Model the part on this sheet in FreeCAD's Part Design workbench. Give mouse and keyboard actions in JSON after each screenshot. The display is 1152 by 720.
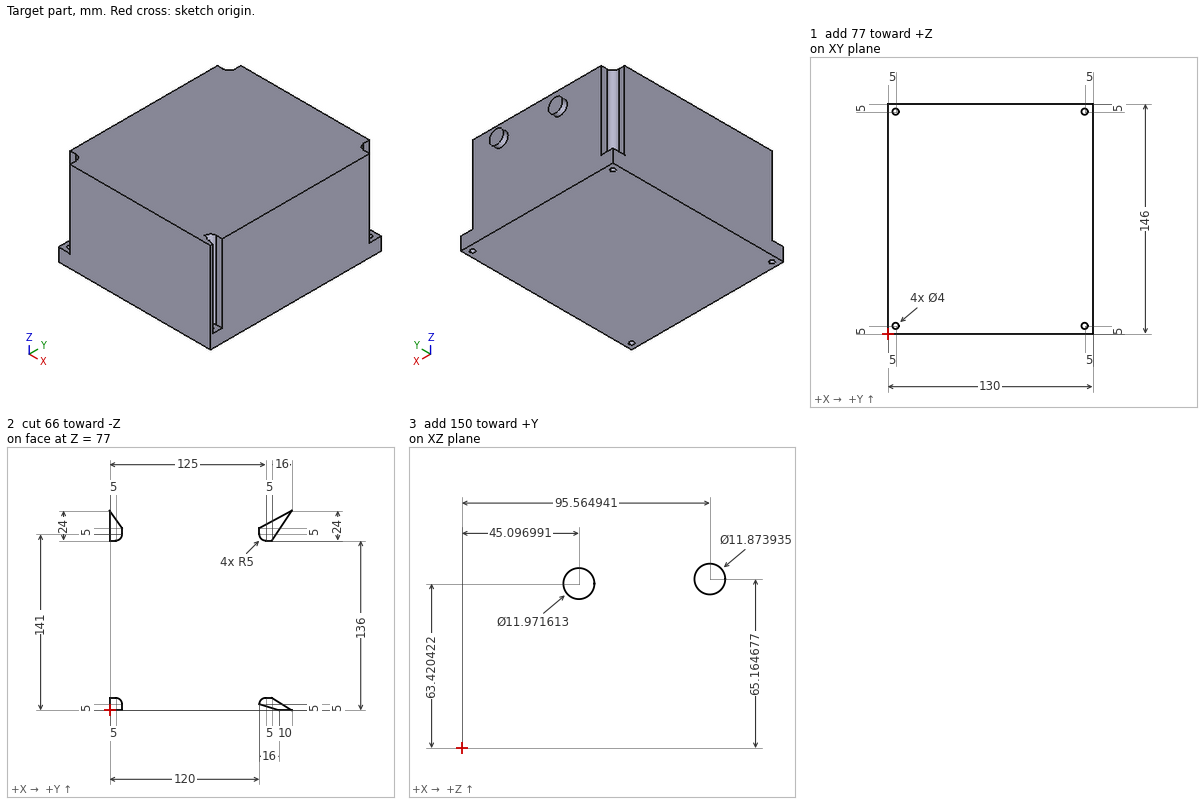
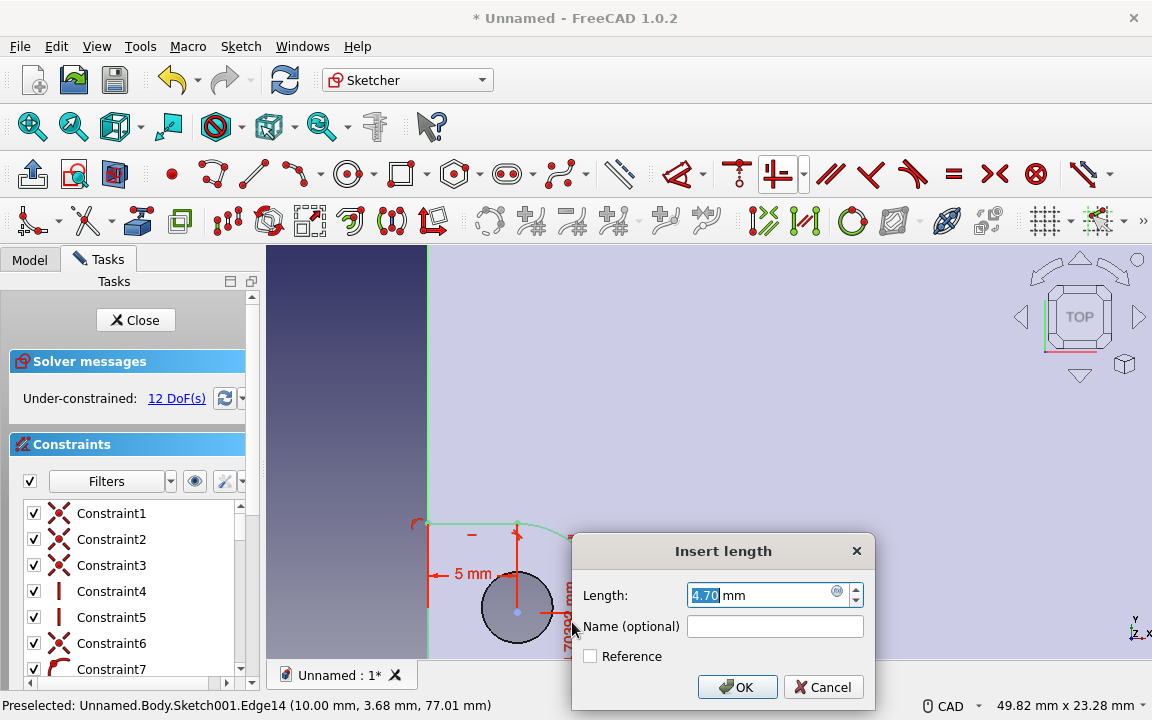
{"action": "type", "text": "5"}
{"action": "key", "text": "Return"}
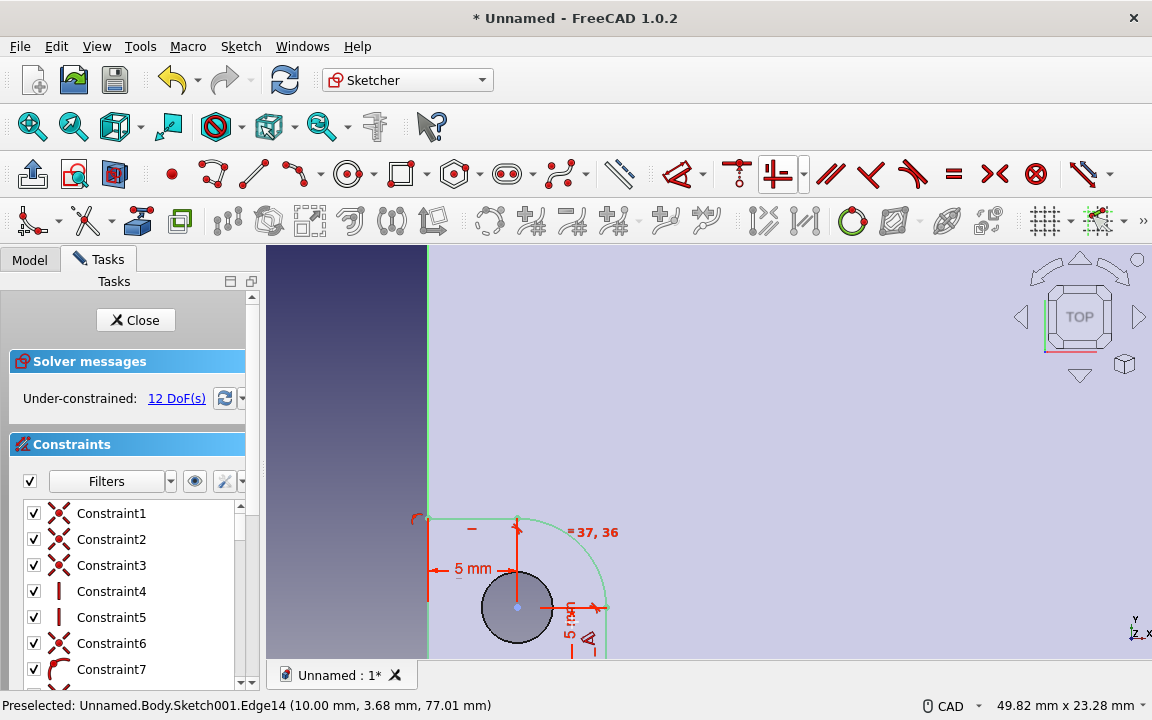
{"action": "scroll", "coordinate": [532, 570], "scroll_direction": "down", "scroll_amount": 12}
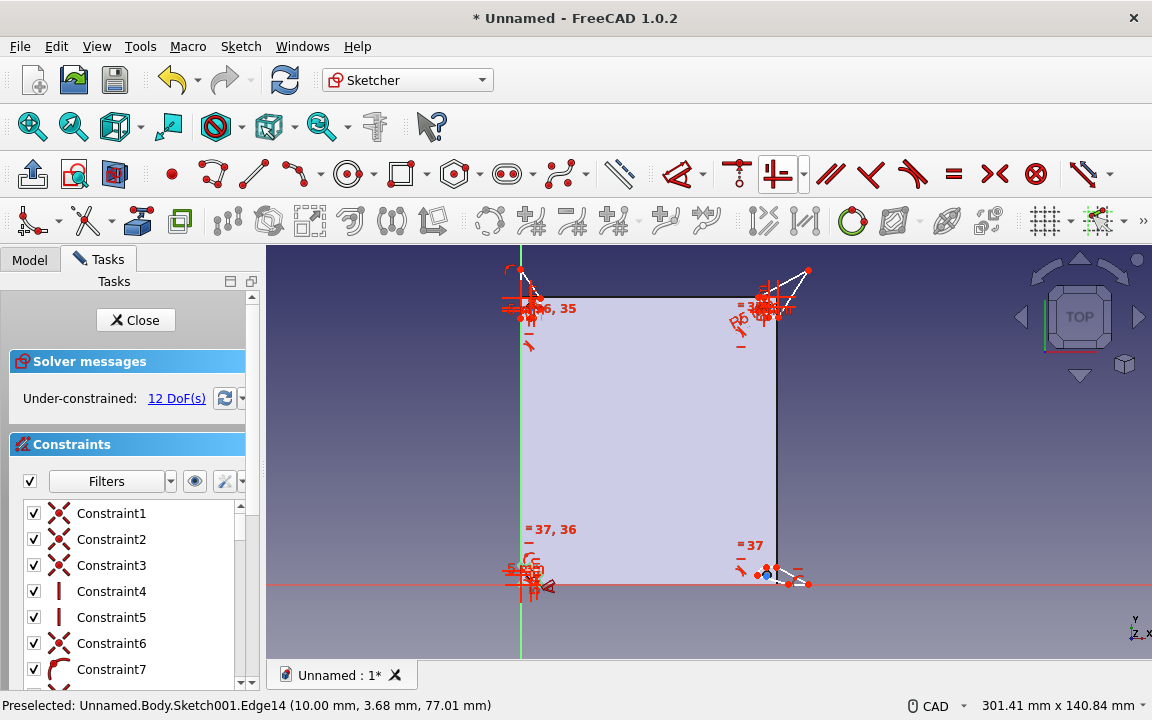
{"action": "scroll", "coordinate": [730, 568], "scroll_direction": "up", "scroll_amount": 9}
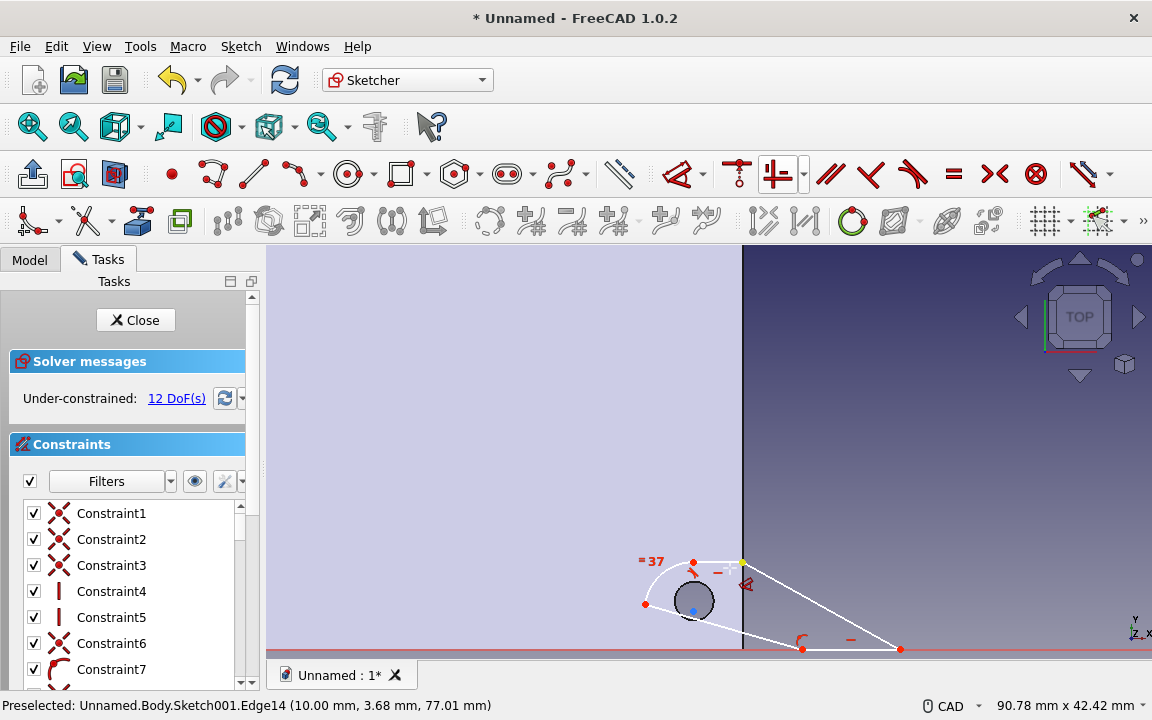
{"action": "left_click", "coordinate": [728, 562]}
{"action": "left_click", "coordinate": [718, 596]}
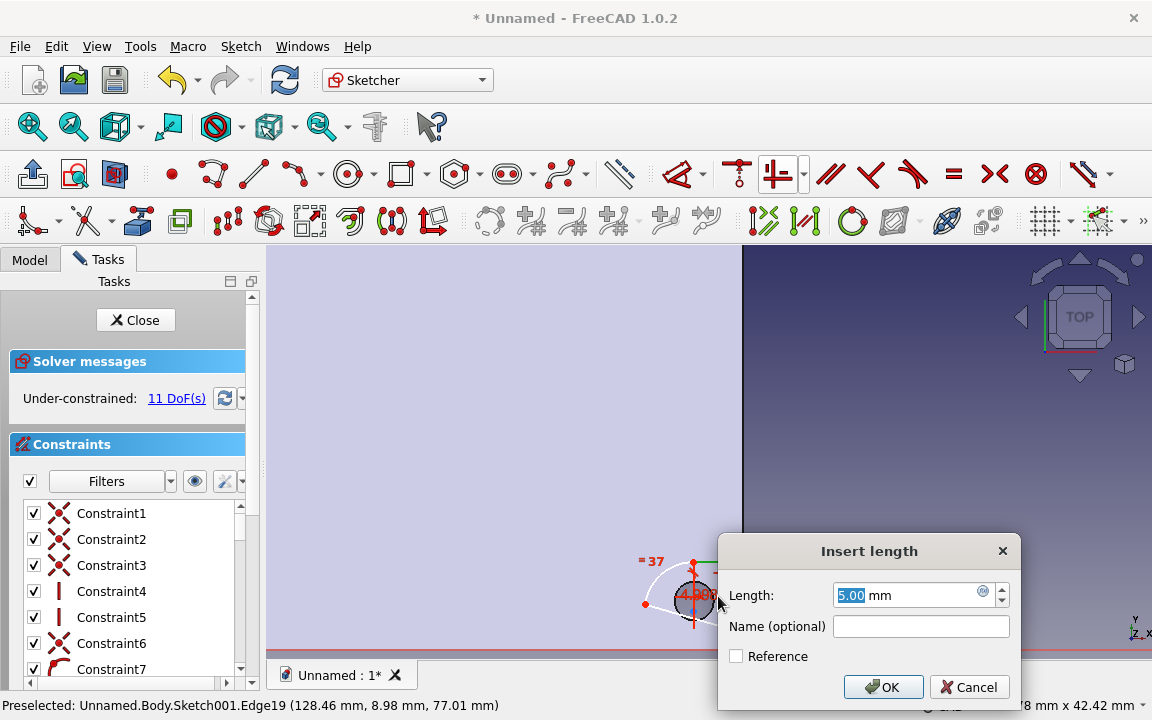
{"action": "type", "text": "5"}
{"action": "key", "text": "Return"}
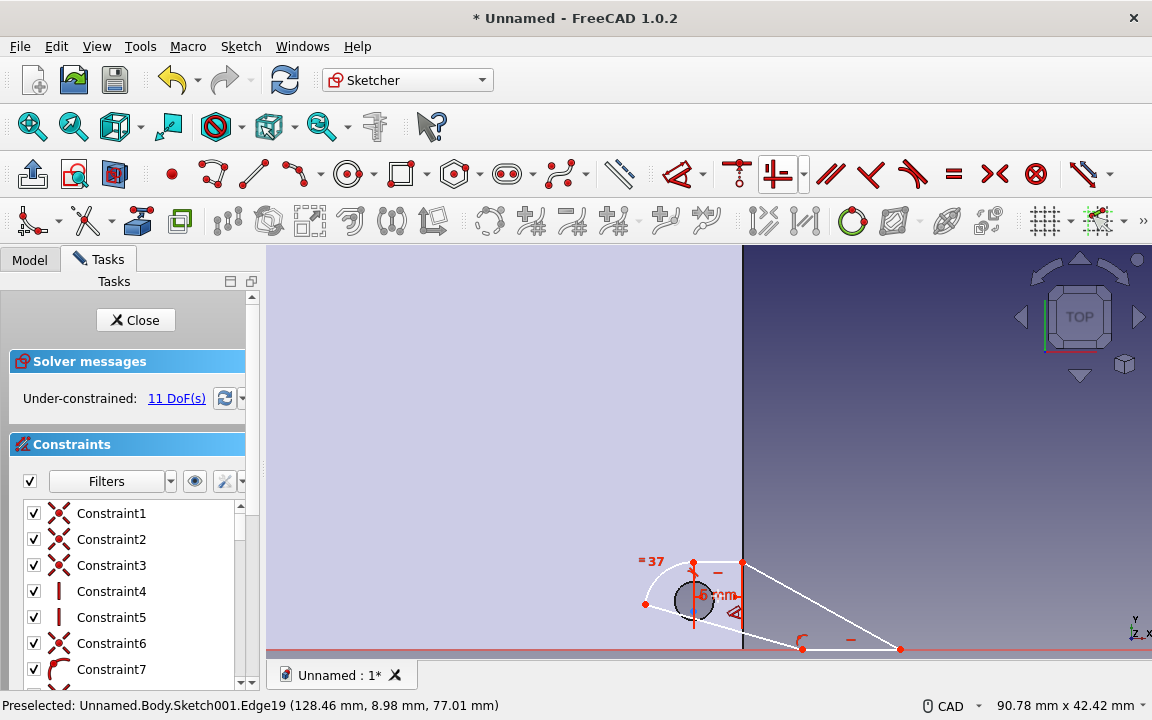
{"action": "scroll", "coordinate": [730, 567], "scroll_direction": "down", "scroll_amount": 9}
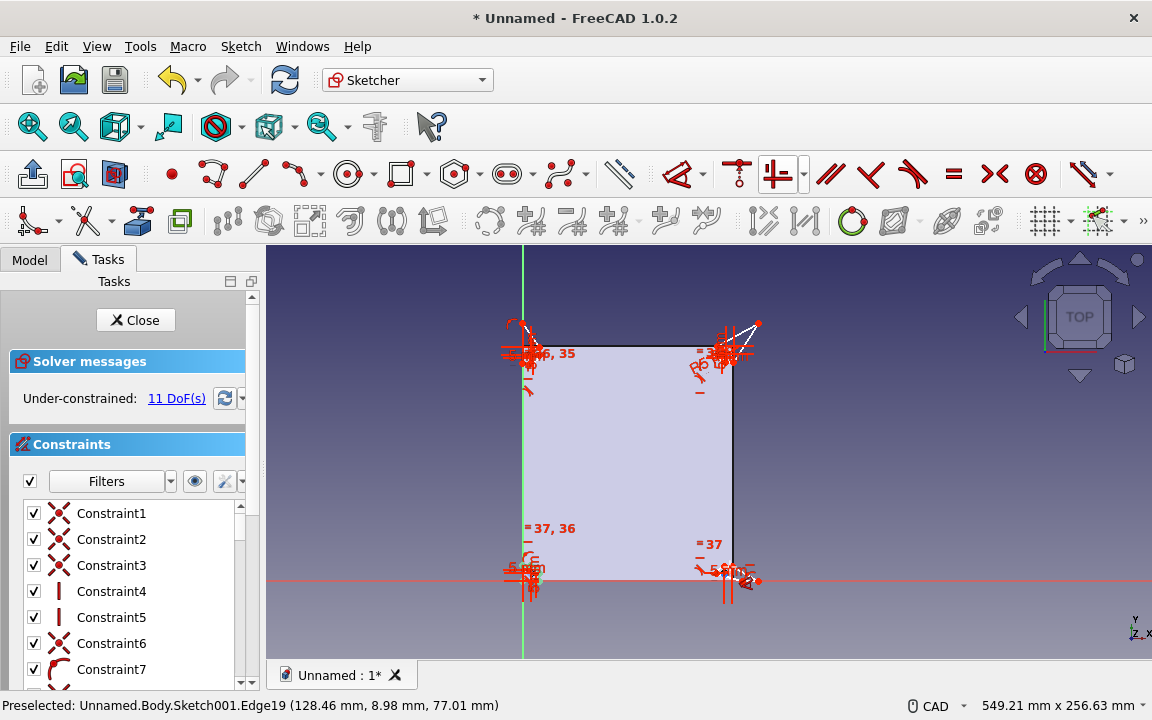
{"action": "scroll", "coordinate": [523, 335], "scroll_direction": "up", "scroll_amount": 4}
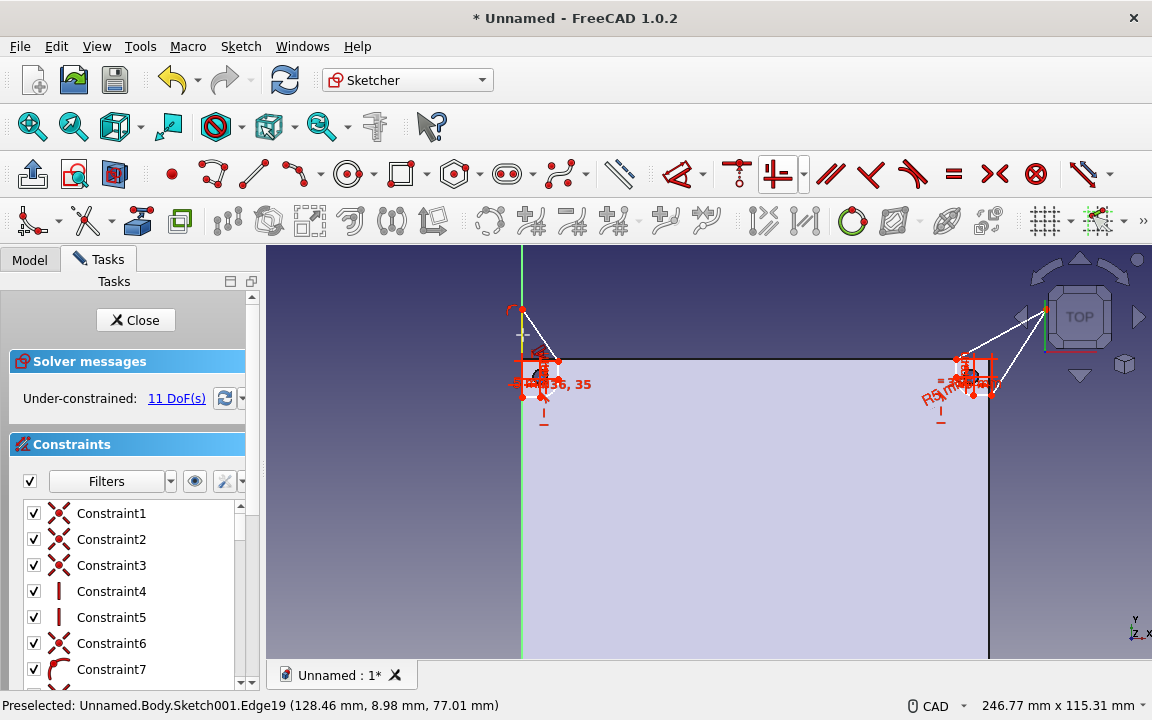
{"action": "left_click", "coordinate": [522, 336]}
{"action": "left_click", "coordinate": [488, 333]}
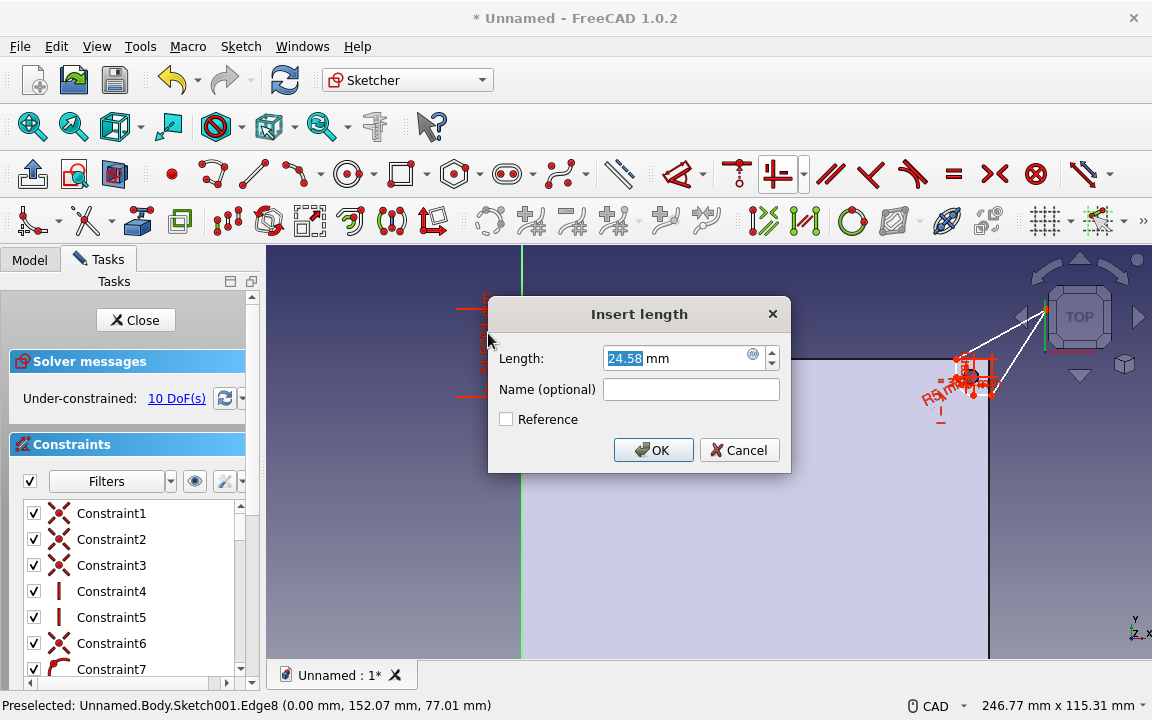
{"action": "type", "text": "24"}
{"action": "key", "text": "Return"}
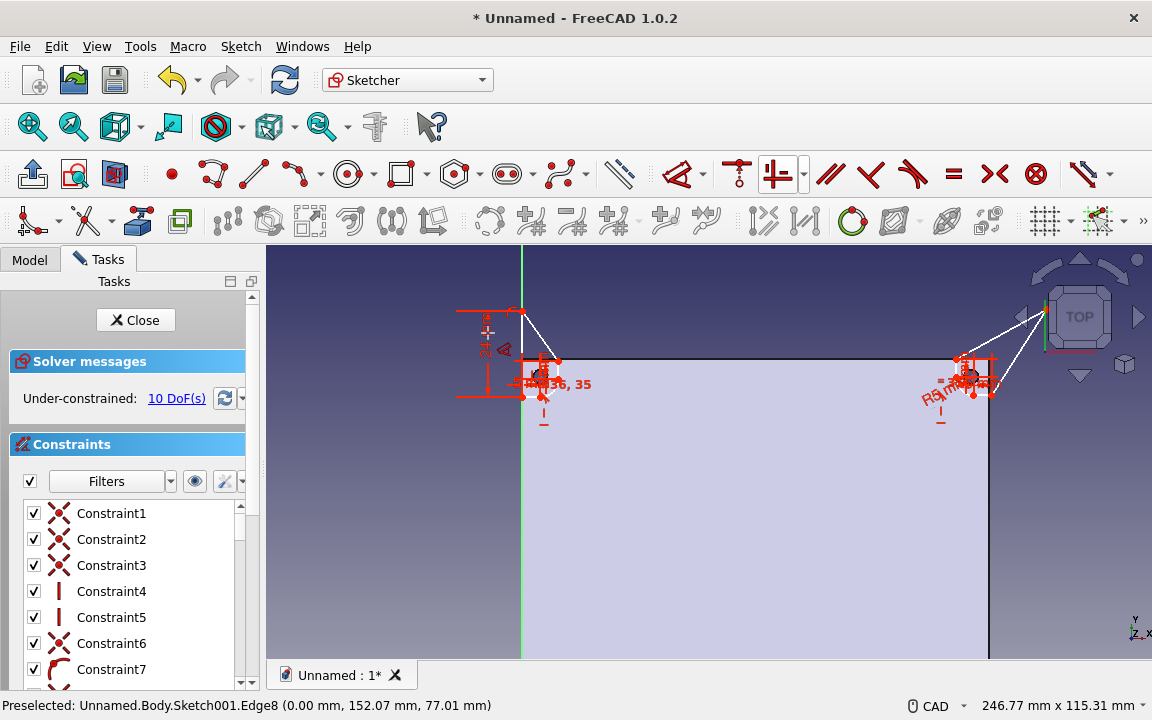
{"action": "scroll", "coordinate": [523, 335], "scroll_direction": "down", "scroll_amount": 4}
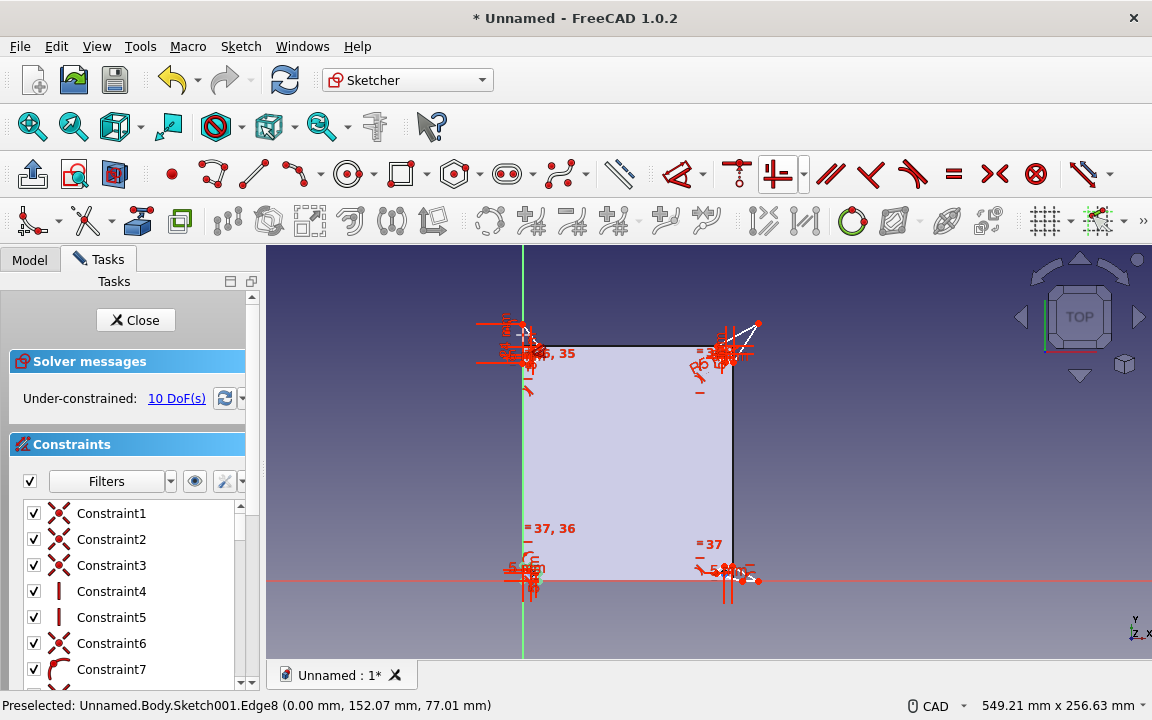
{"action": "scroll", "coordinate": [747, 581], "scroll_direction": "up", "scroll_amount": 6}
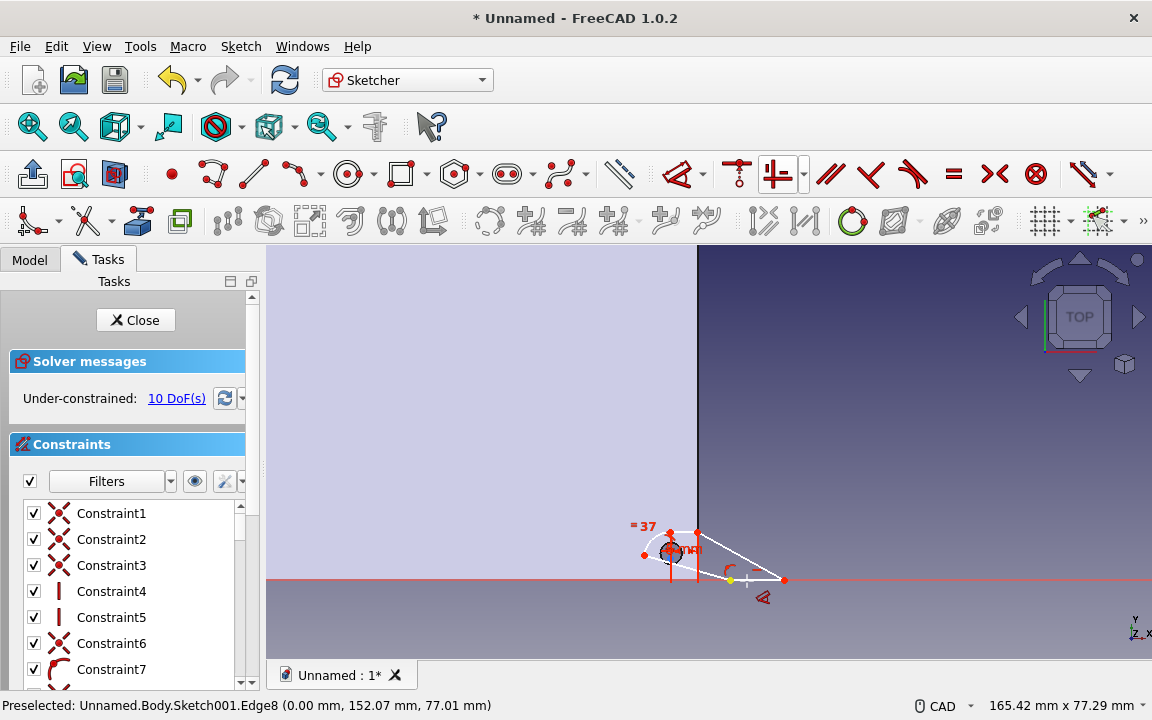
{"action": "left_click", "coordinate": [747, 580]}
{"action": "left_click", "coordinate": [757, 614]}